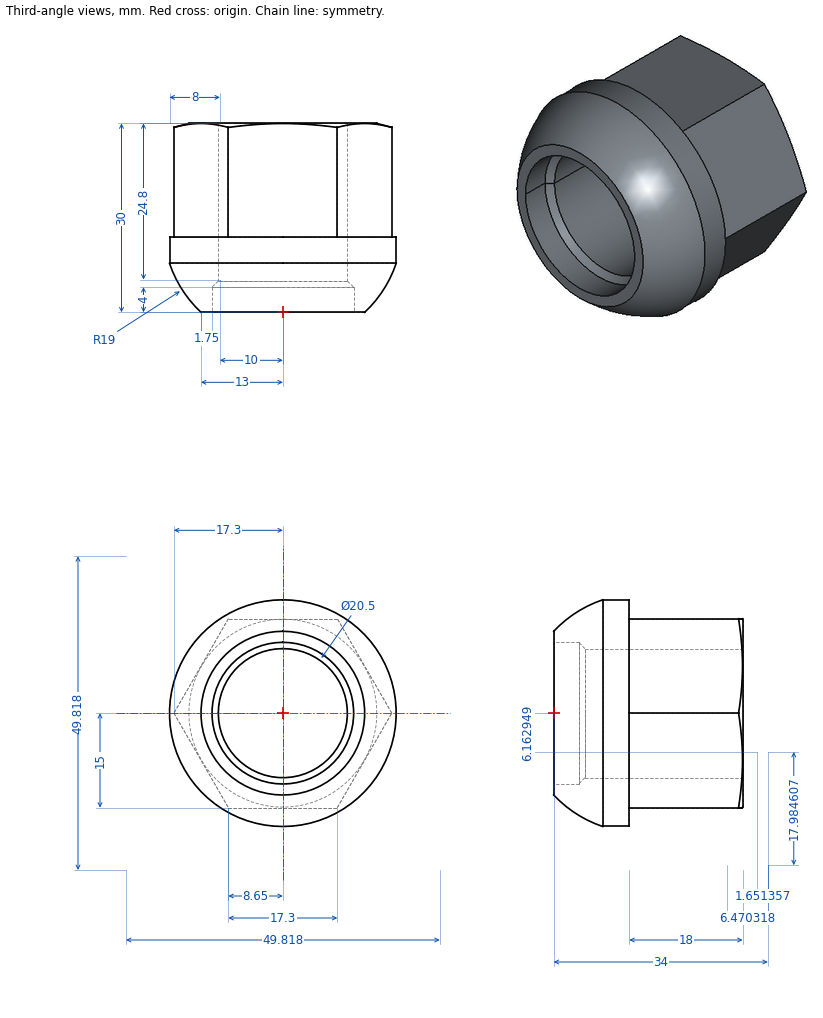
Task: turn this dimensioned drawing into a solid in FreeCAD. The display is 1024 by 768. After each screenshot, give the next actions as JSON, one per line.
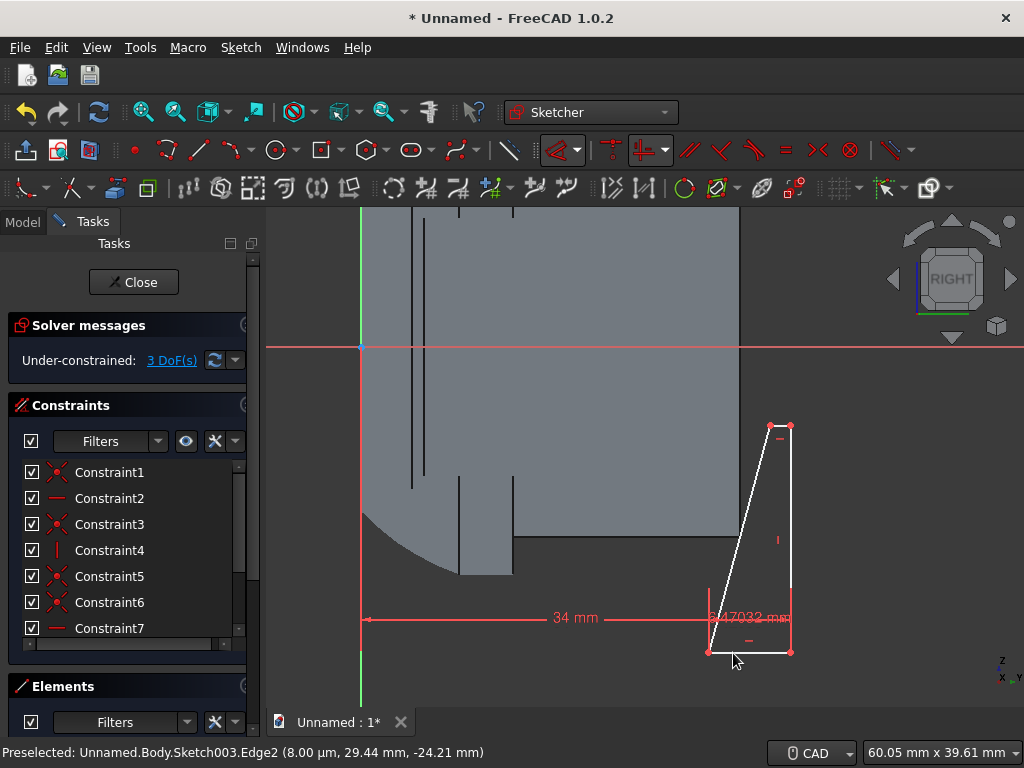
{"action": "scroll", "coordinate": [780, 426], "scroll_direction": "up", "scroll_amount": 4}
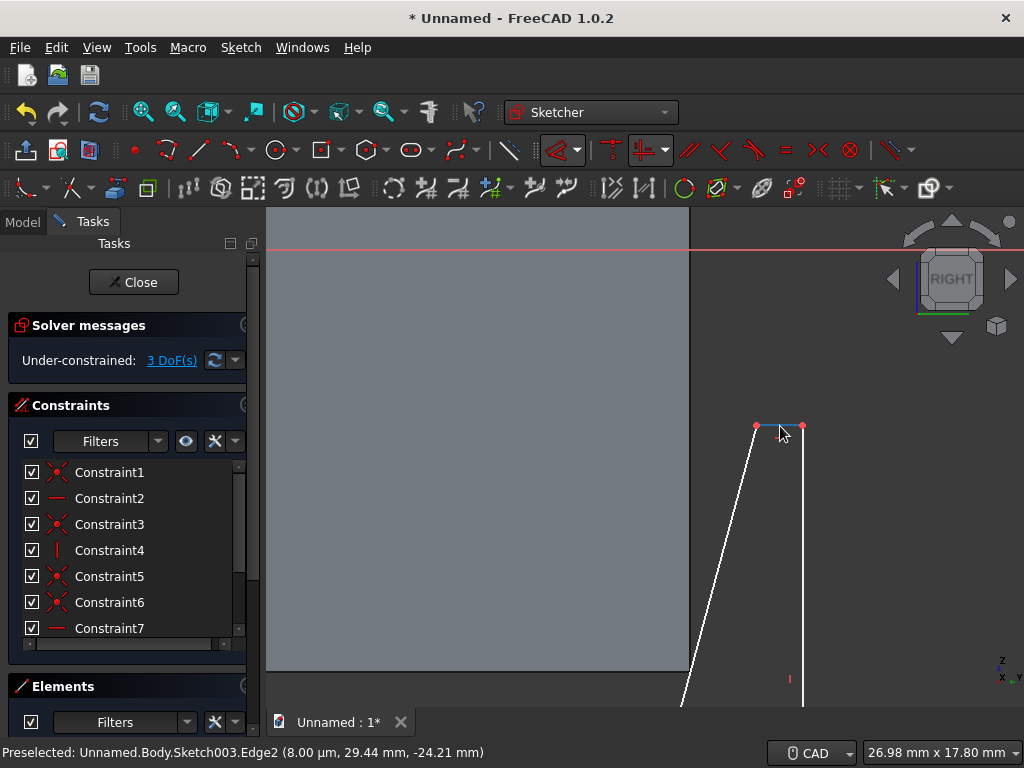
{"action": "left_click", "coordinate": [780, 425]}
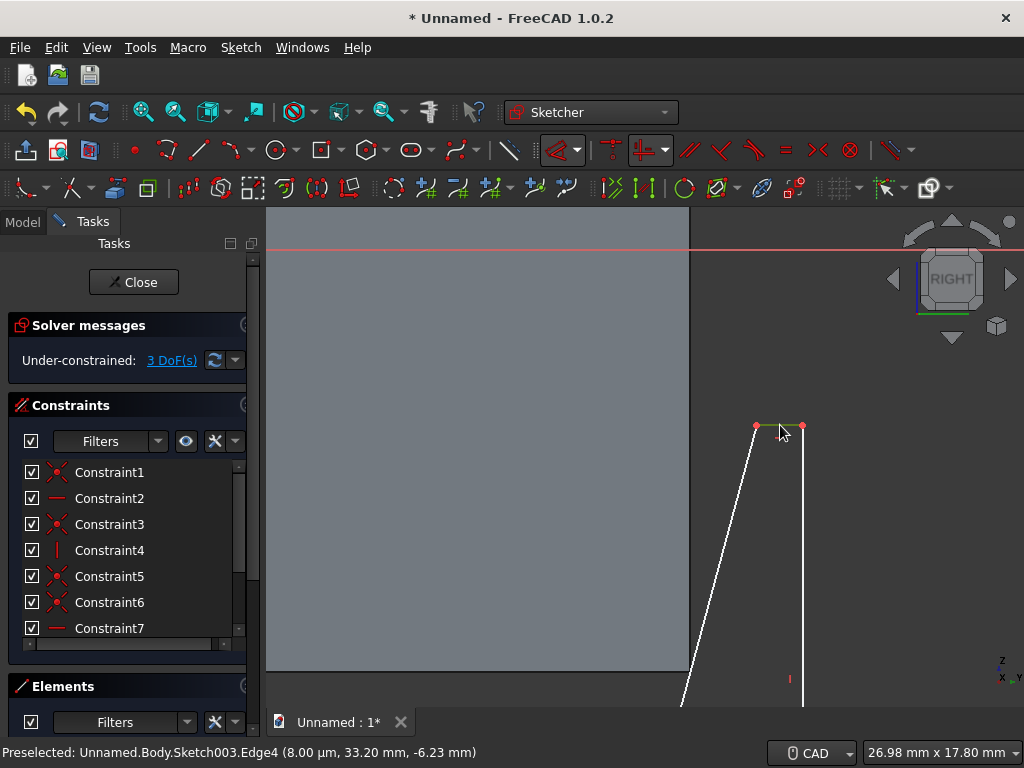
{"action": "key", "text": "l"}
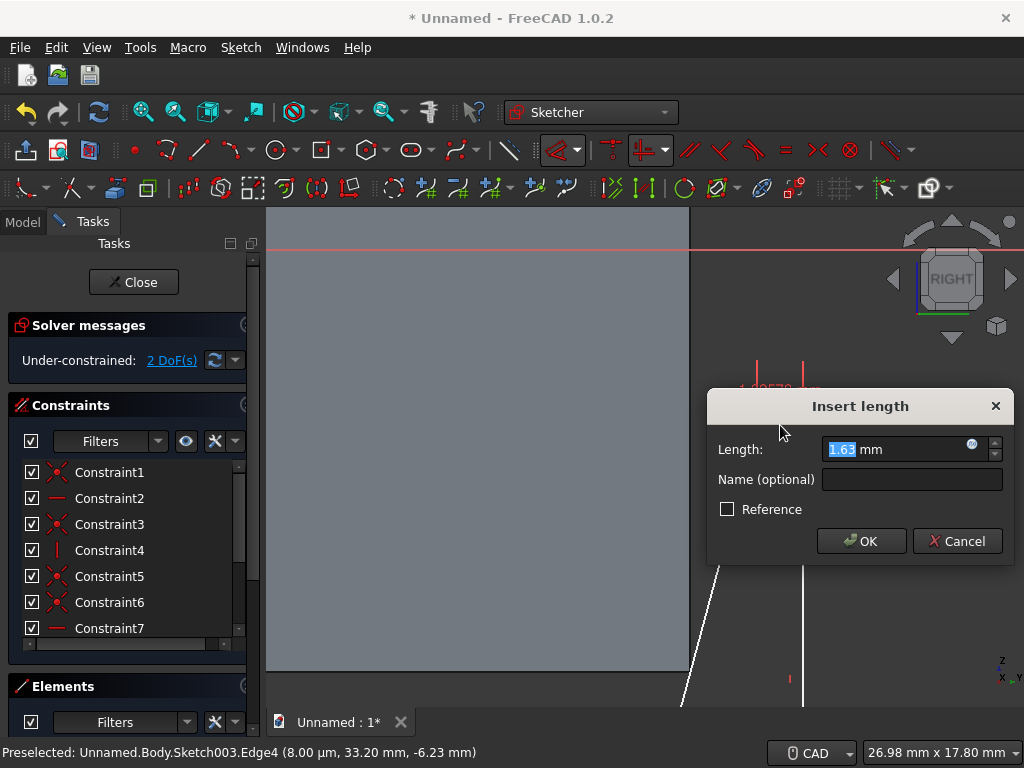
{"action": "type", "text": "1.651357"}
{"action": "key", "text": "Return"}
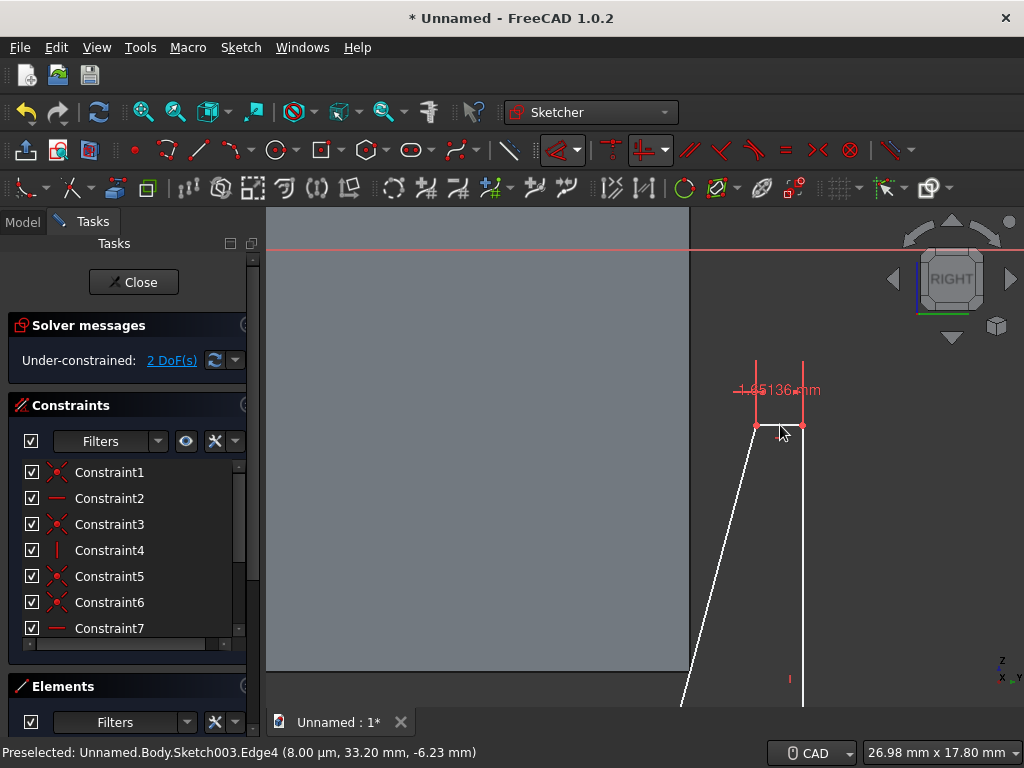
{"action": "left_click", "coordinate": [803, 577]}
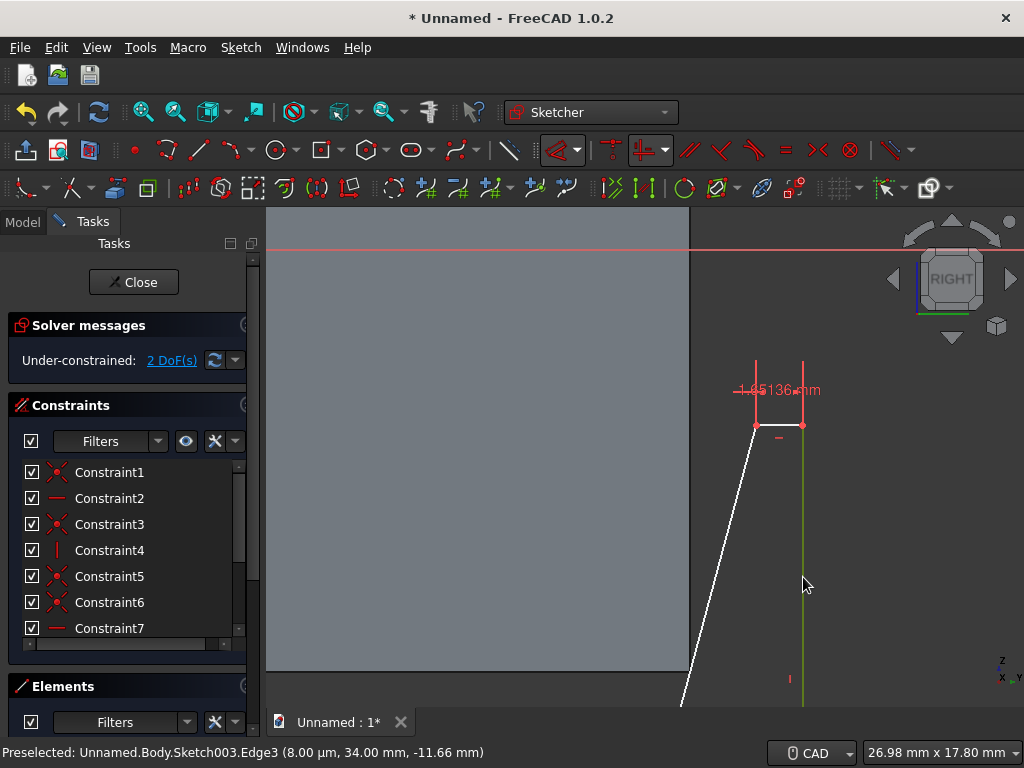
{"action": "key", "text": "i"}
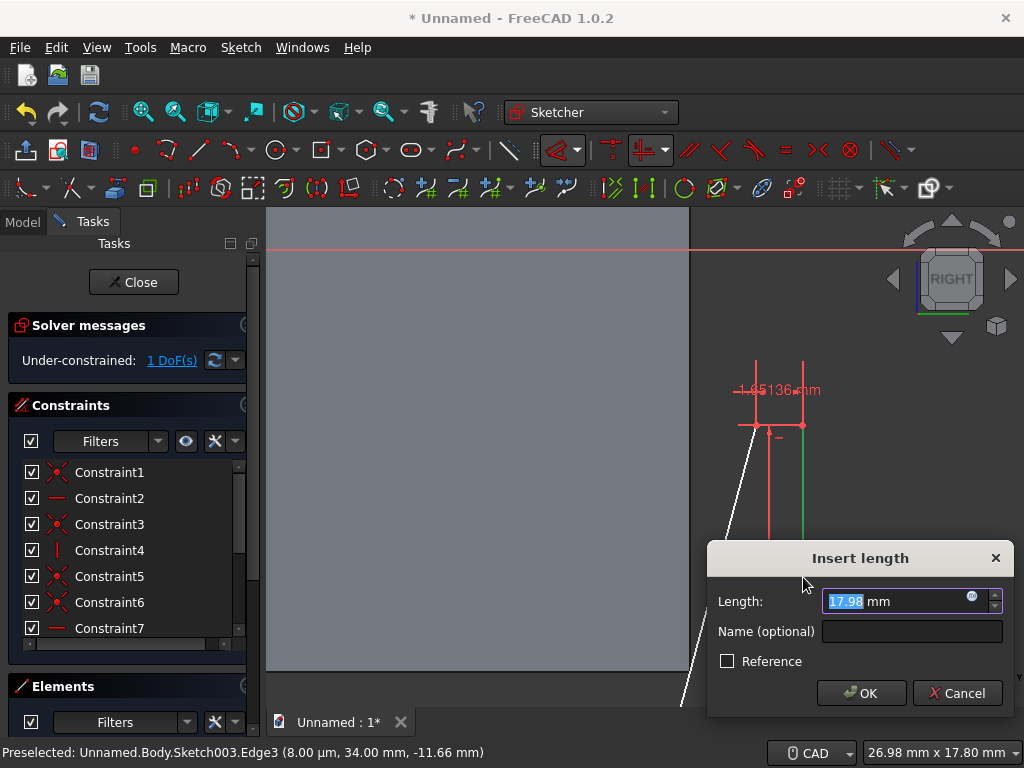
{"action": "type", "text": "17.984607"}
{"action": "key", "text": "Return"}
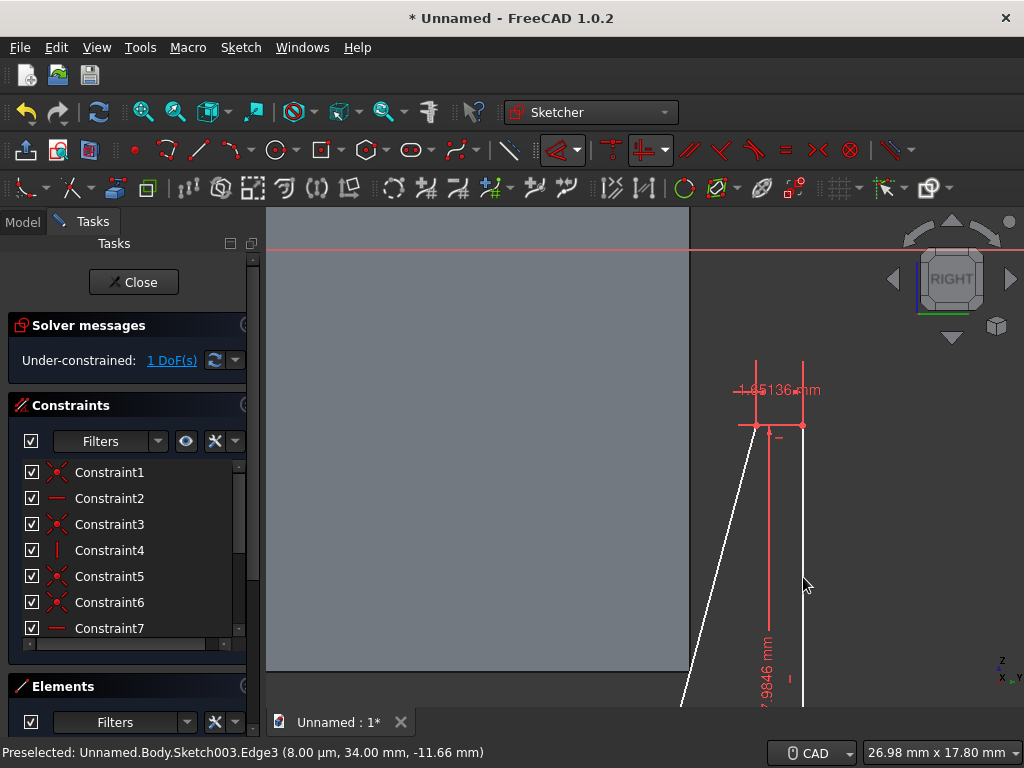
{"action": "left_click", "coordinate": [756, 425]}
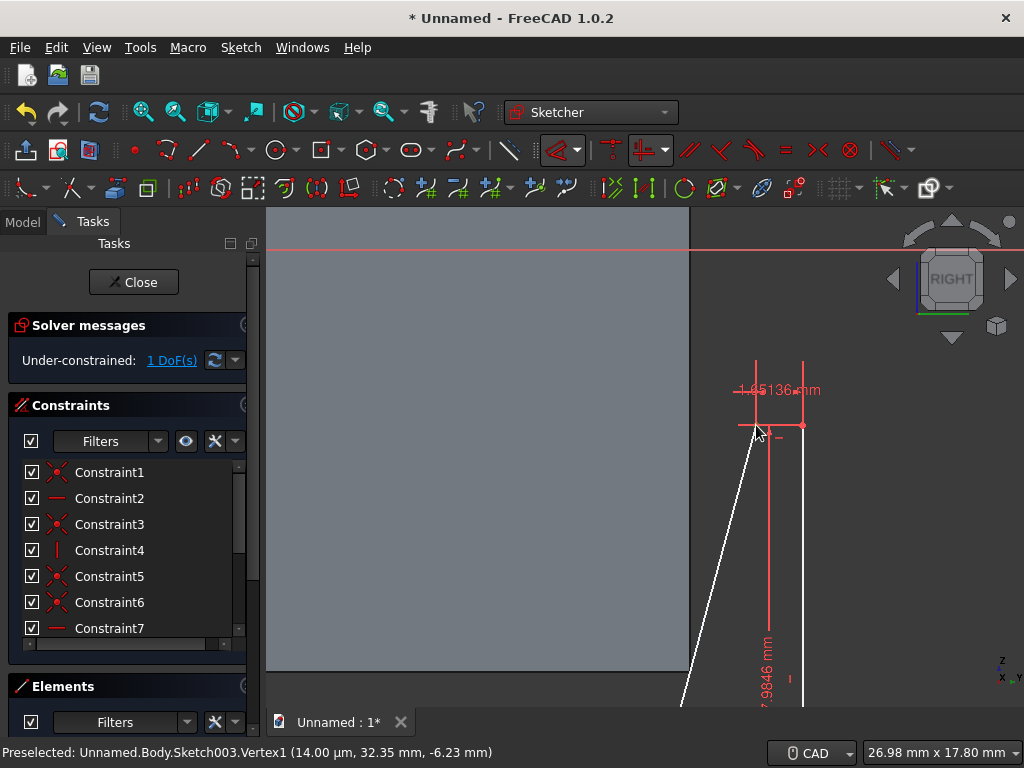
{"action": "key", "text": "i"}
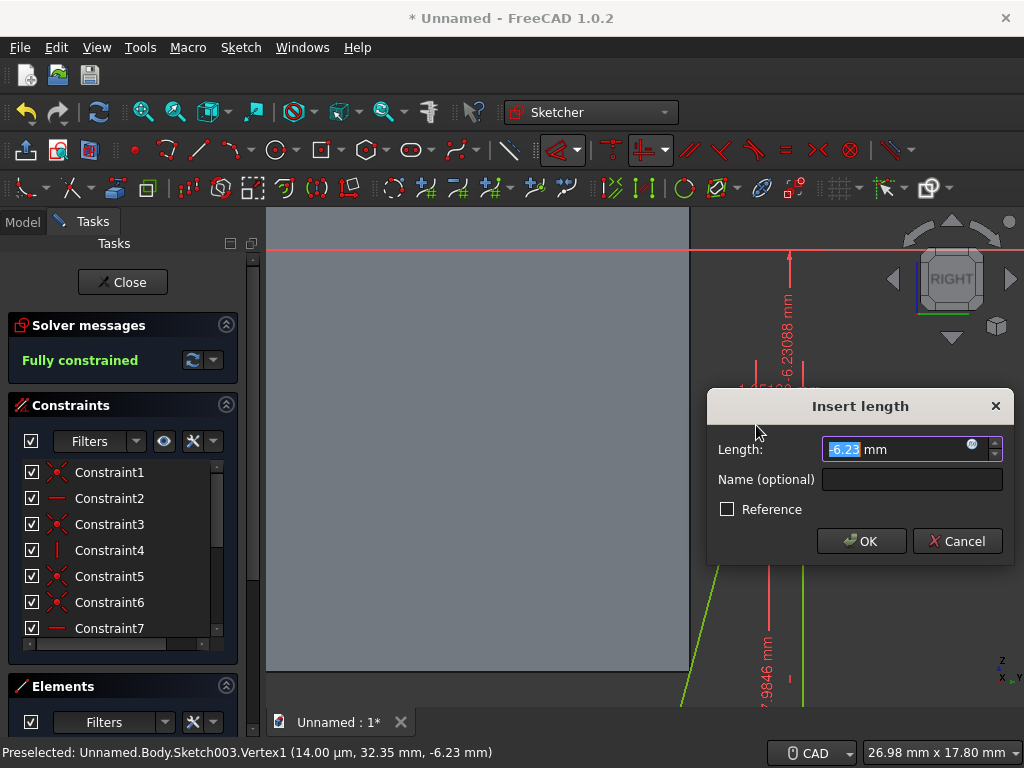
{"action": "type", "text": "-6.162949"}
{"action": "key", "text": "Return"}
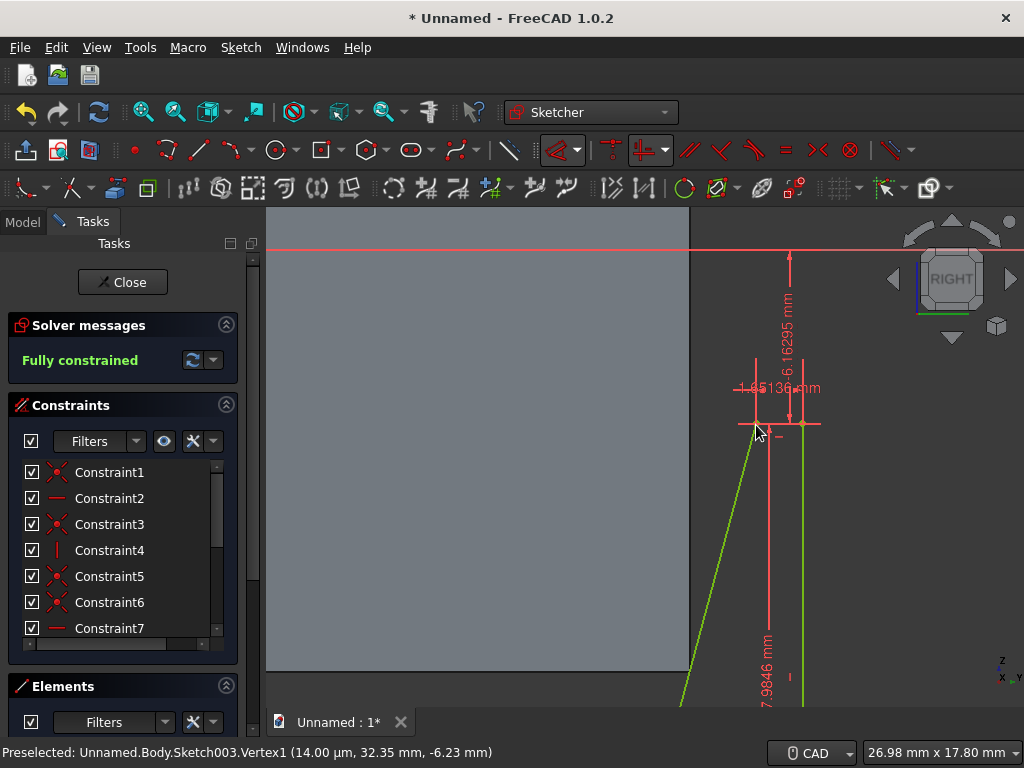
{"action": "left_click", "coordinate": [123, 282]}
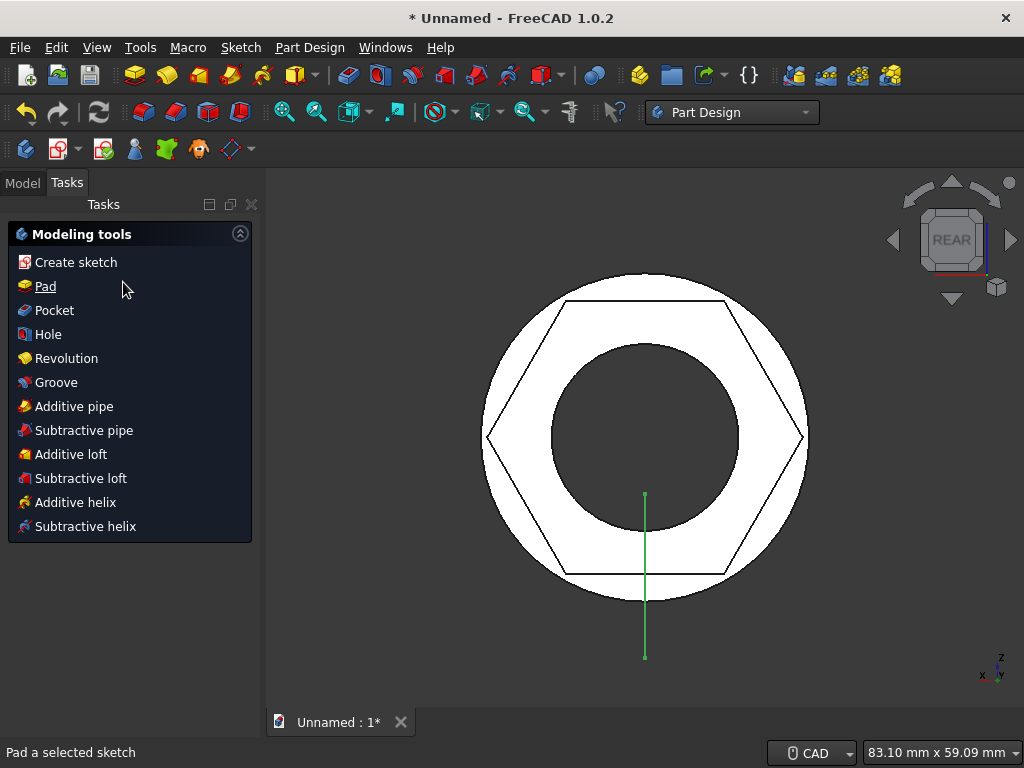
{"action": "left_click", "coordinate": [414, 76]}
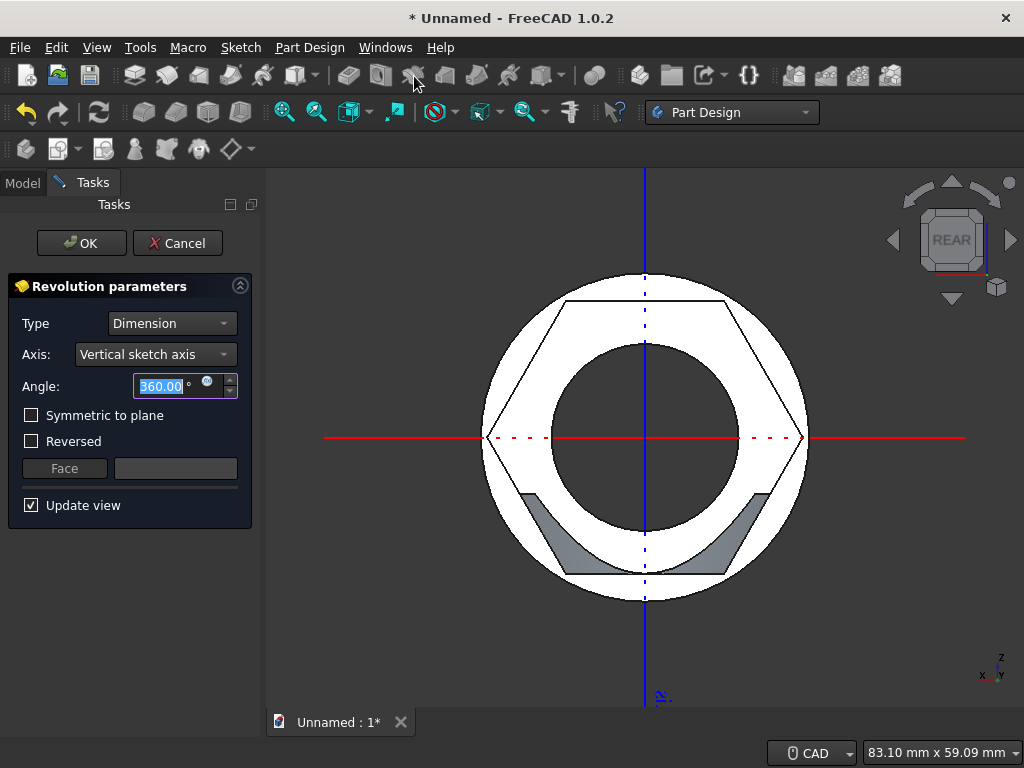
{"action": "left_click", "coordinate": [156, 354]}